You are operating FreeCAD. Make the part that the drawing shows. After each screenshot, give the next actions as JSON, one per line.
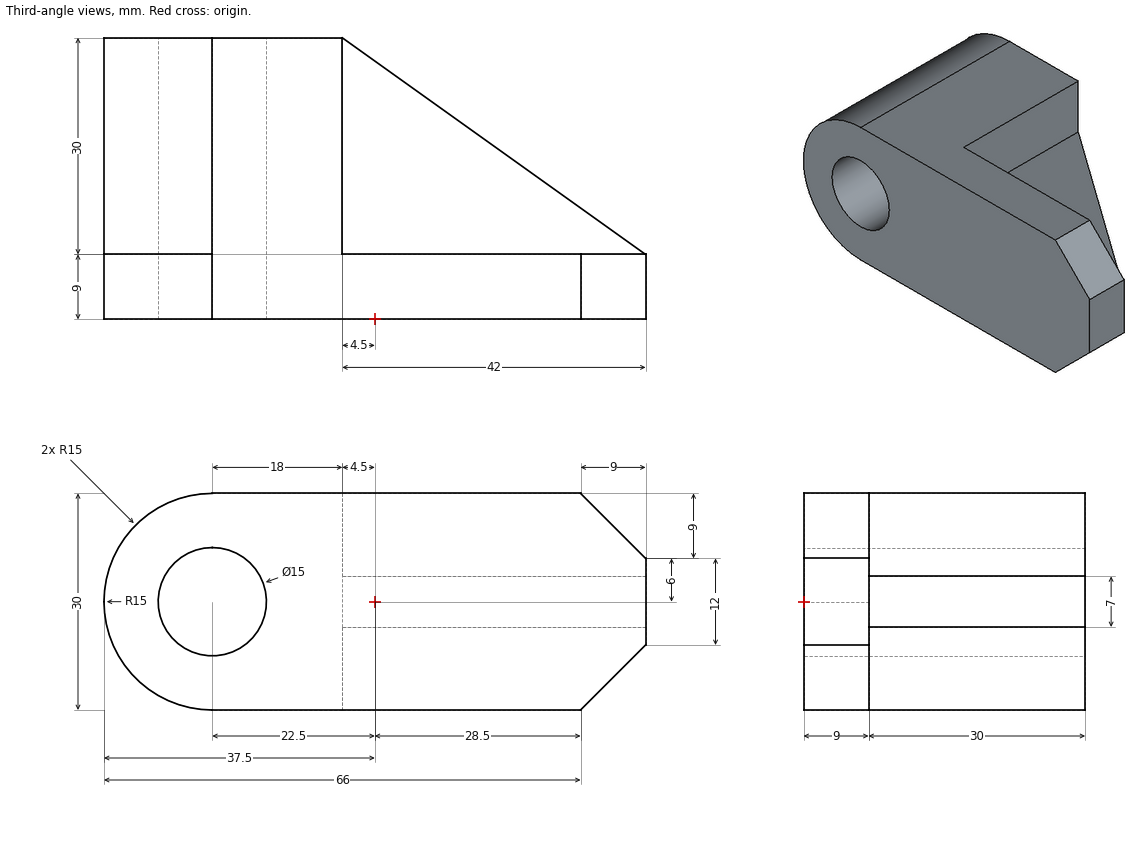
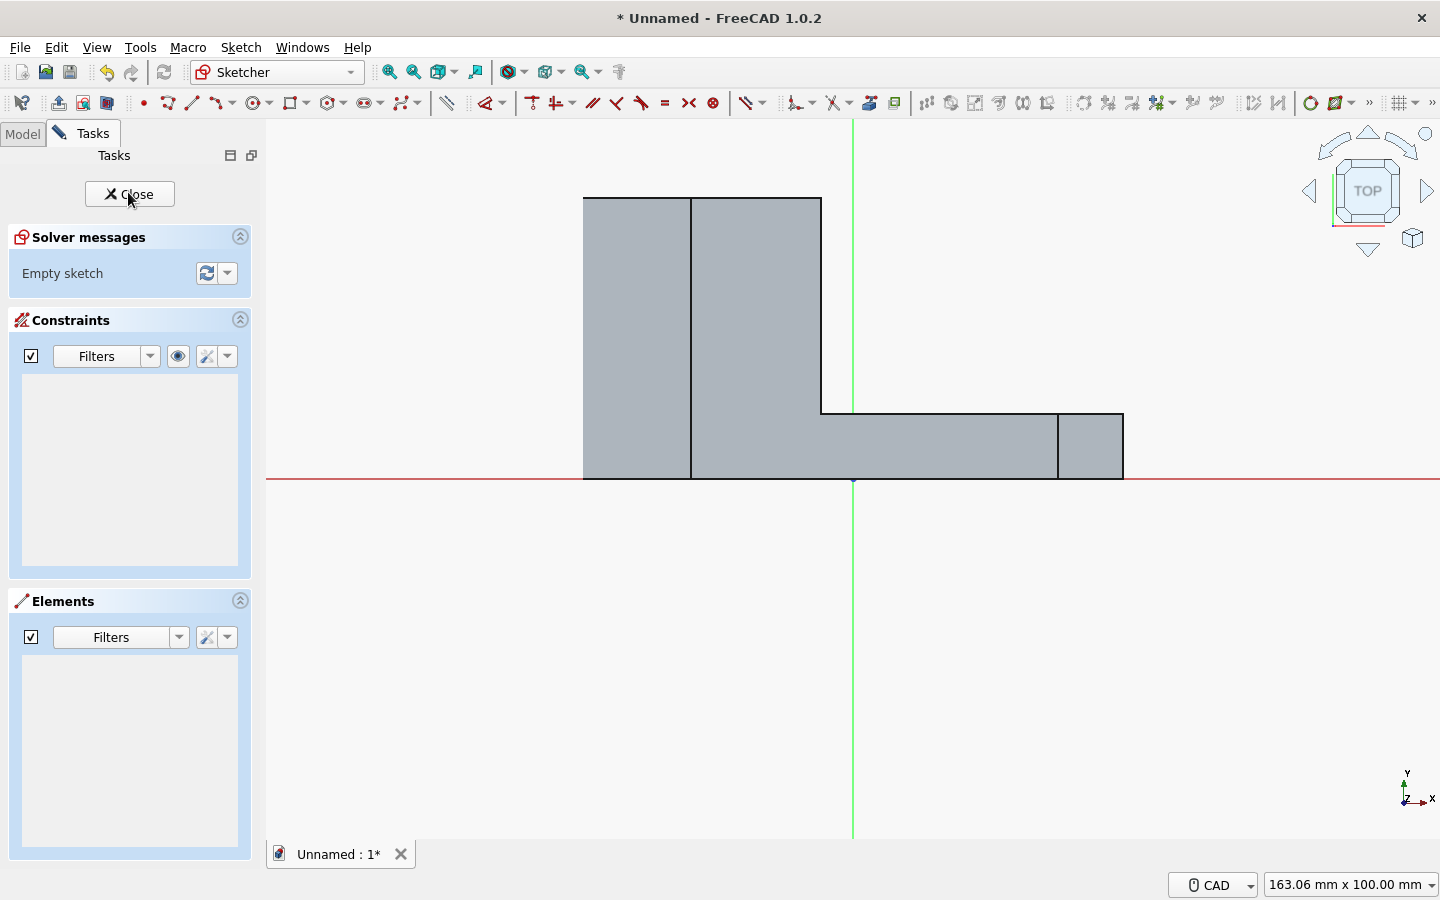
{"action": "key", "text": "q s"}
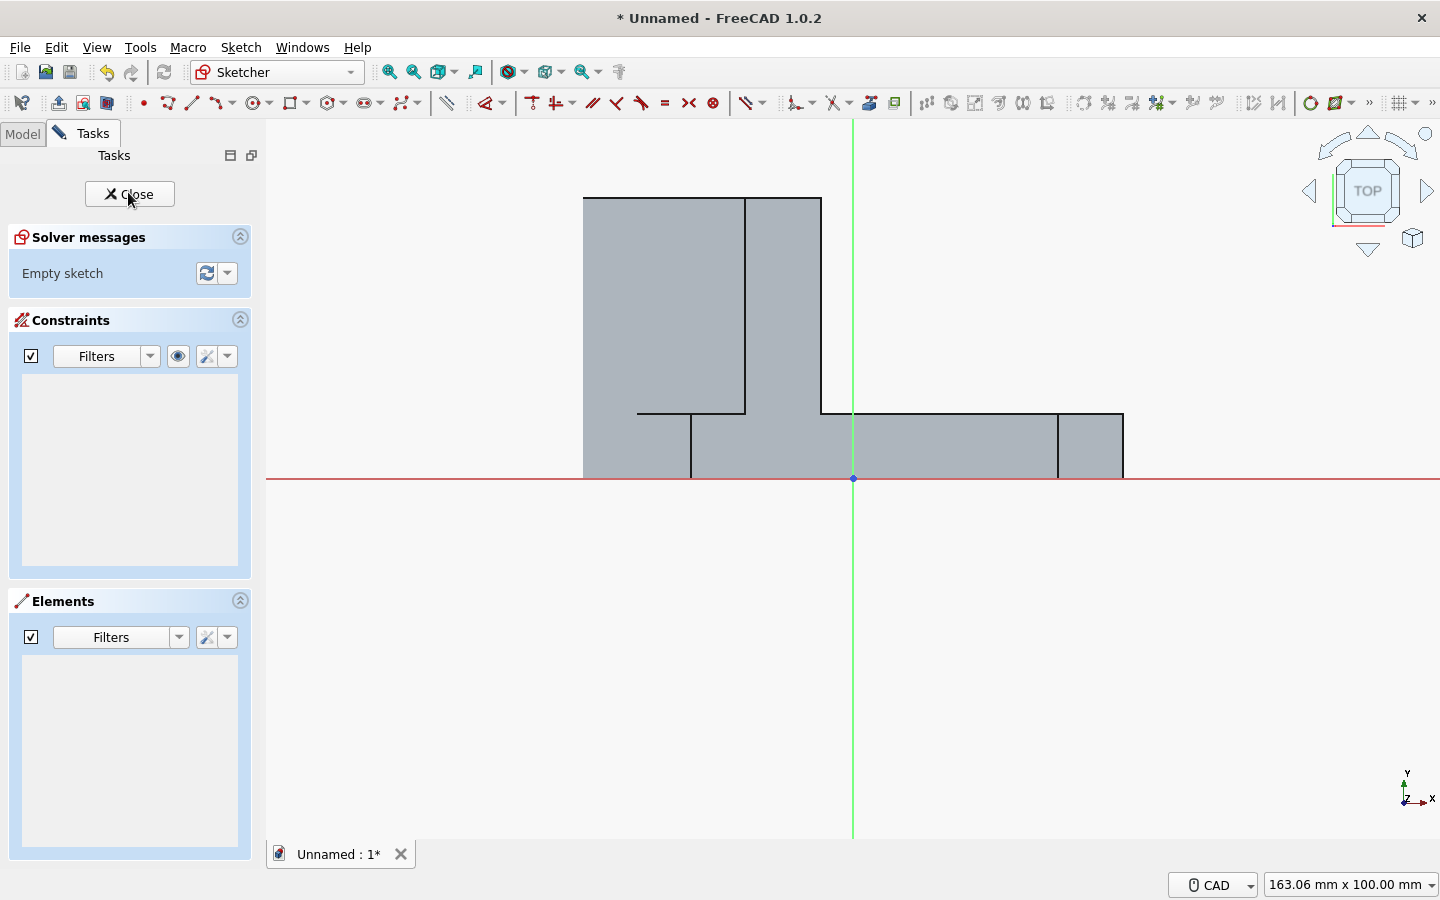
{"action": "scroll", "coordinate": [1200, 168], "scroll_direction": "up", "scroll_amount": 3}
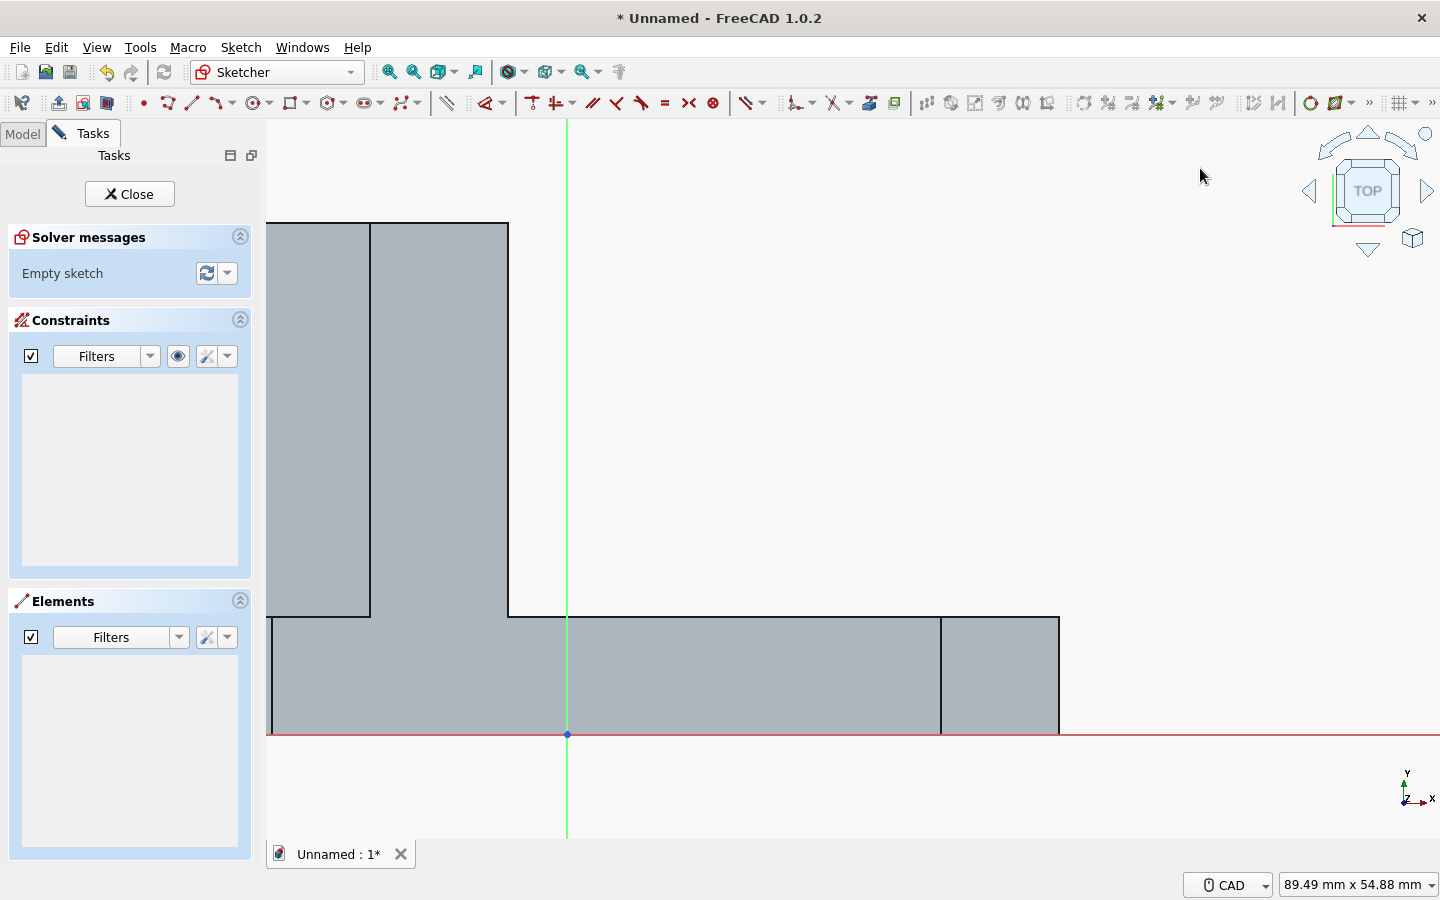
{"action": "left_click", "coordinate": [168, 104]}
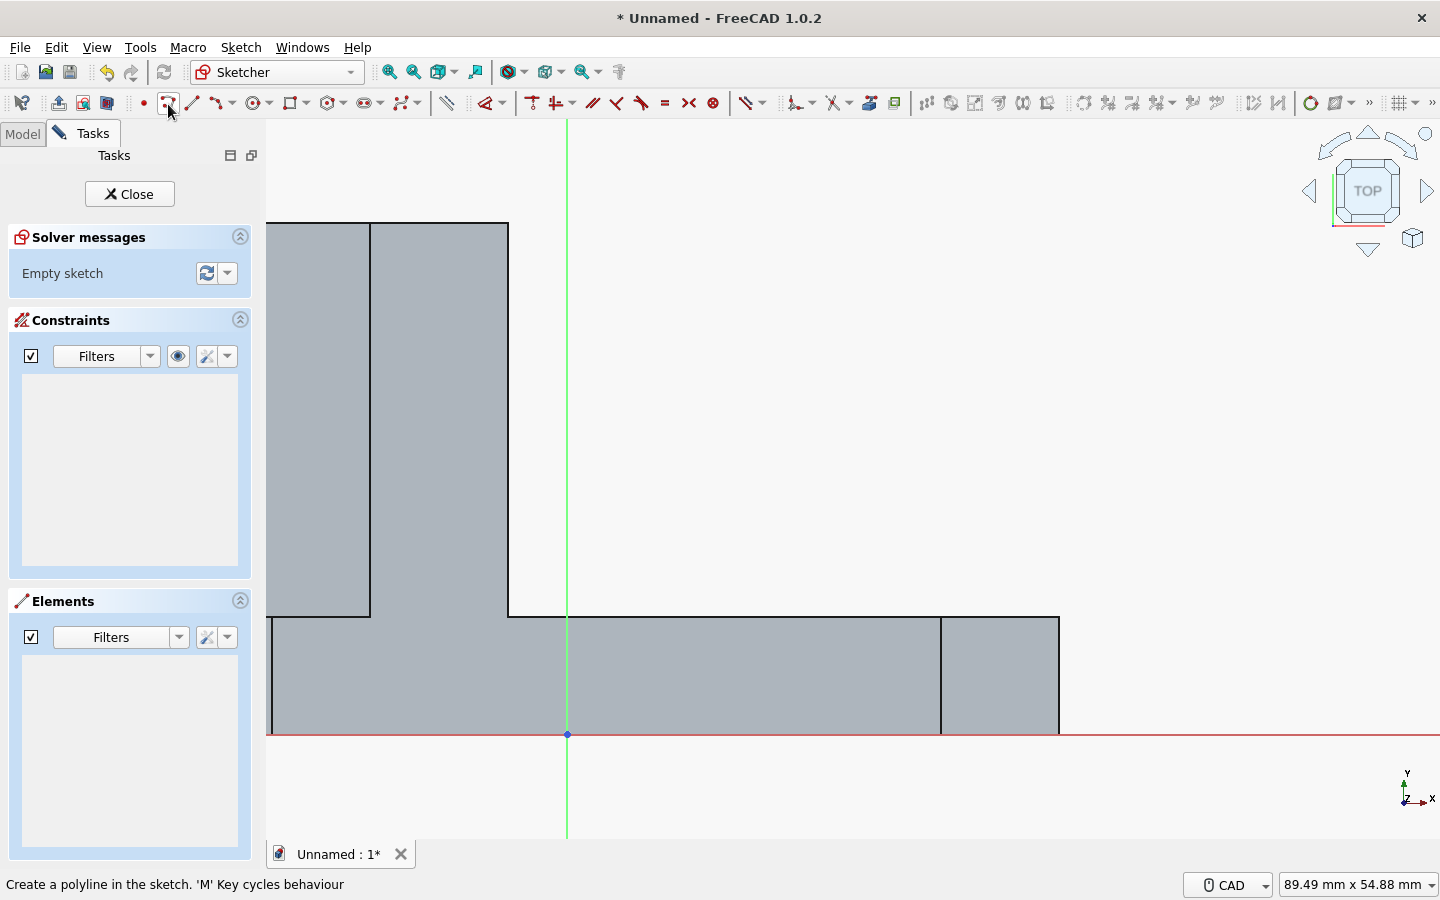
{"action": "left_click", "coordinate": [508, 617]}
{"action": "left_click", "coordinate": [1059, 617]}
{"action": "left_click", "coordinate": [508, 223]}
{"action": "left_click", "coordinate": [508, 618]}
{"action": "key", "text": "Escape"}
{"action": "key", "text": "Escape"}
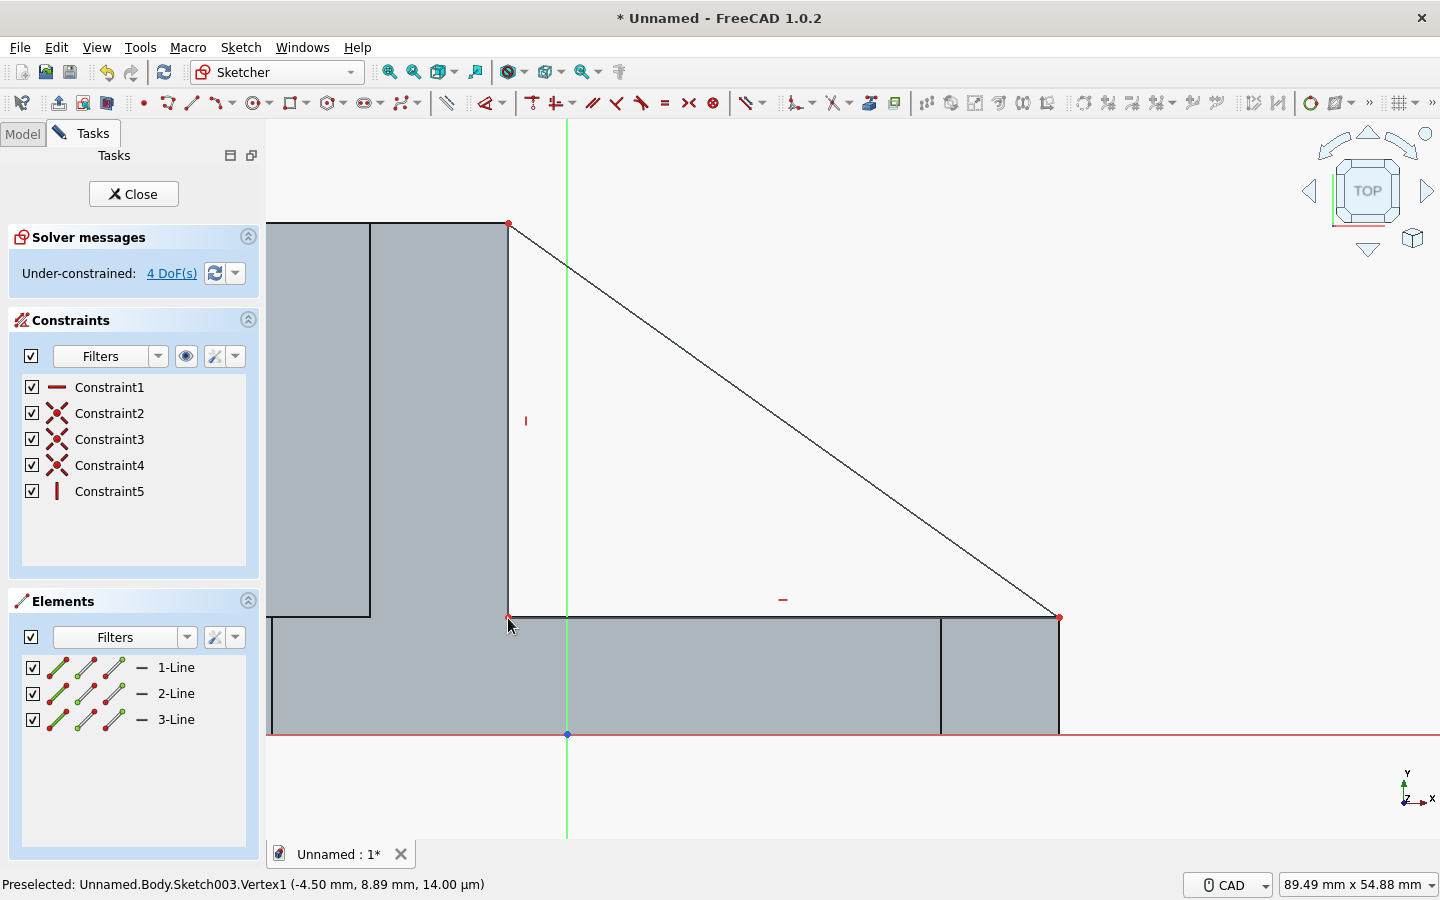
{"action": "key", "text": "d"}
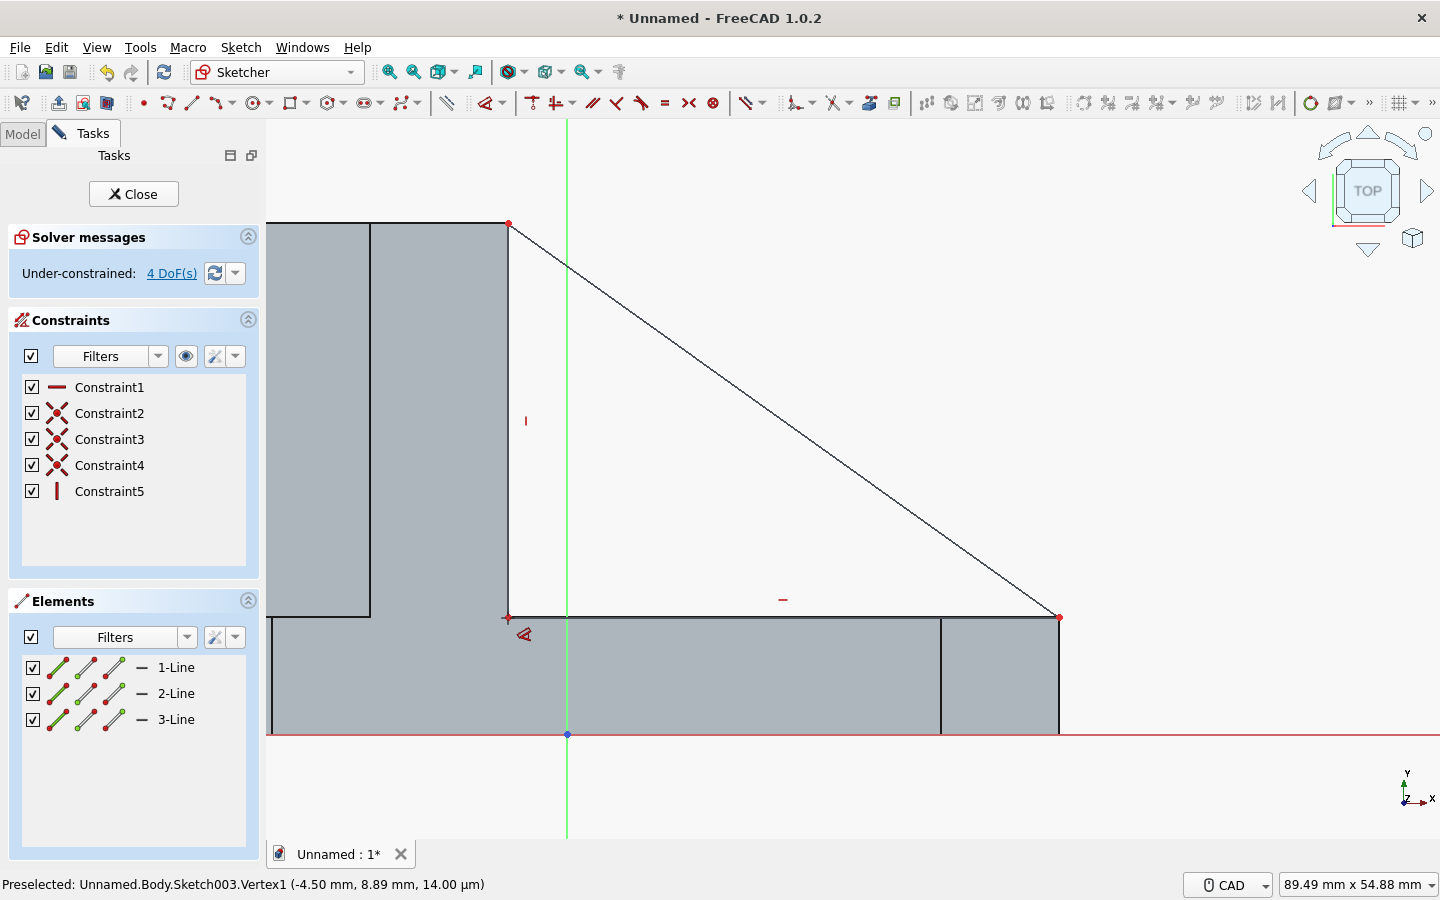
{"action": "left_click", "coordinate": [673, 618]}
{"action": "left_click", "coordinate": [784, 652]}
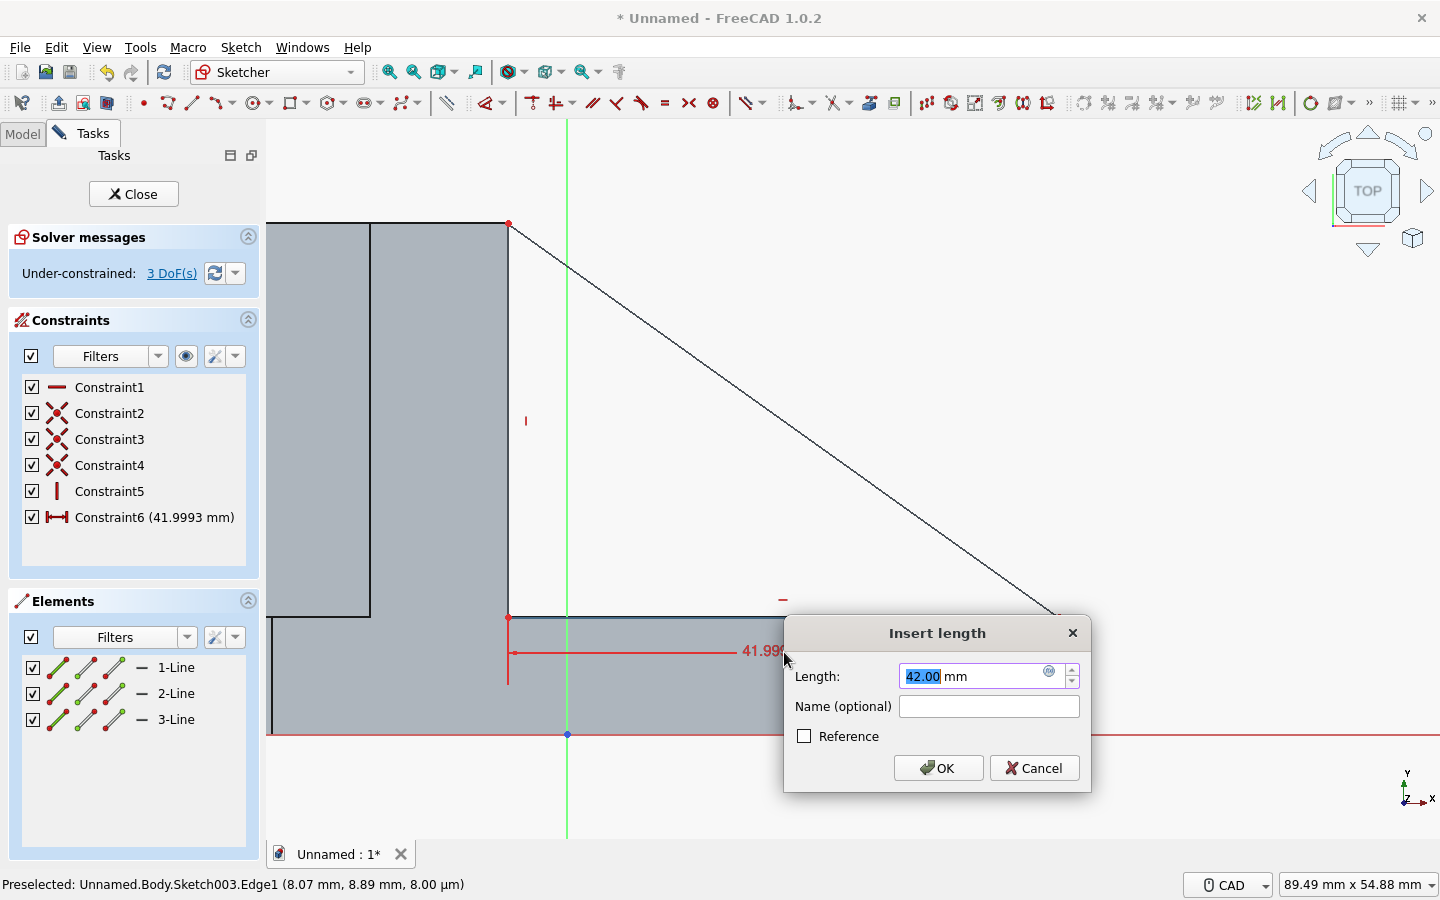
{"action": "type", "text": "42"}
{"action": "key", "text": "Return"}